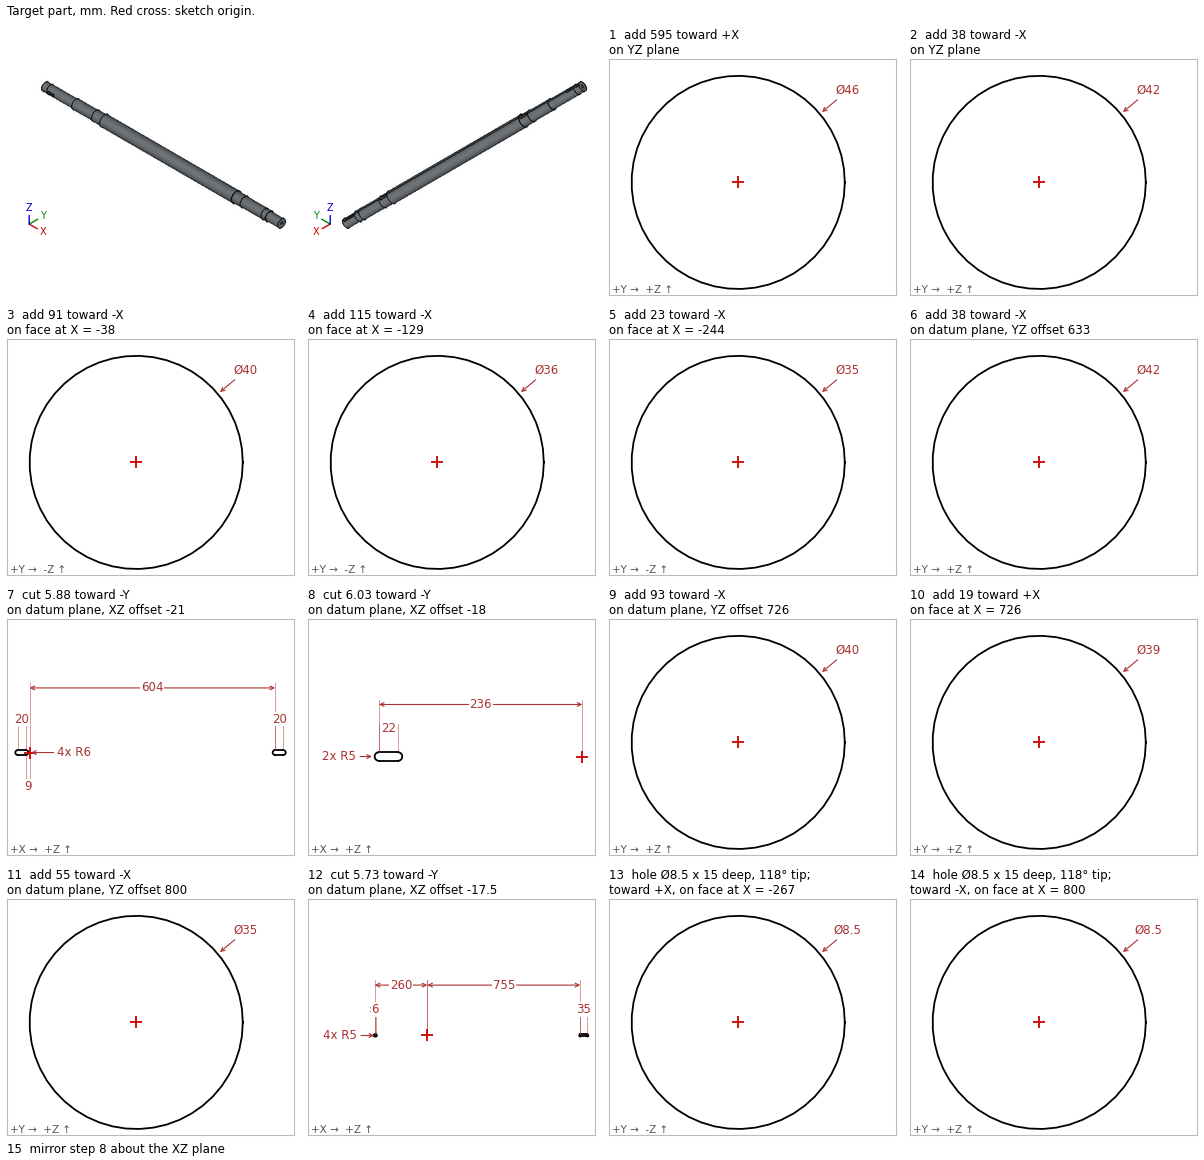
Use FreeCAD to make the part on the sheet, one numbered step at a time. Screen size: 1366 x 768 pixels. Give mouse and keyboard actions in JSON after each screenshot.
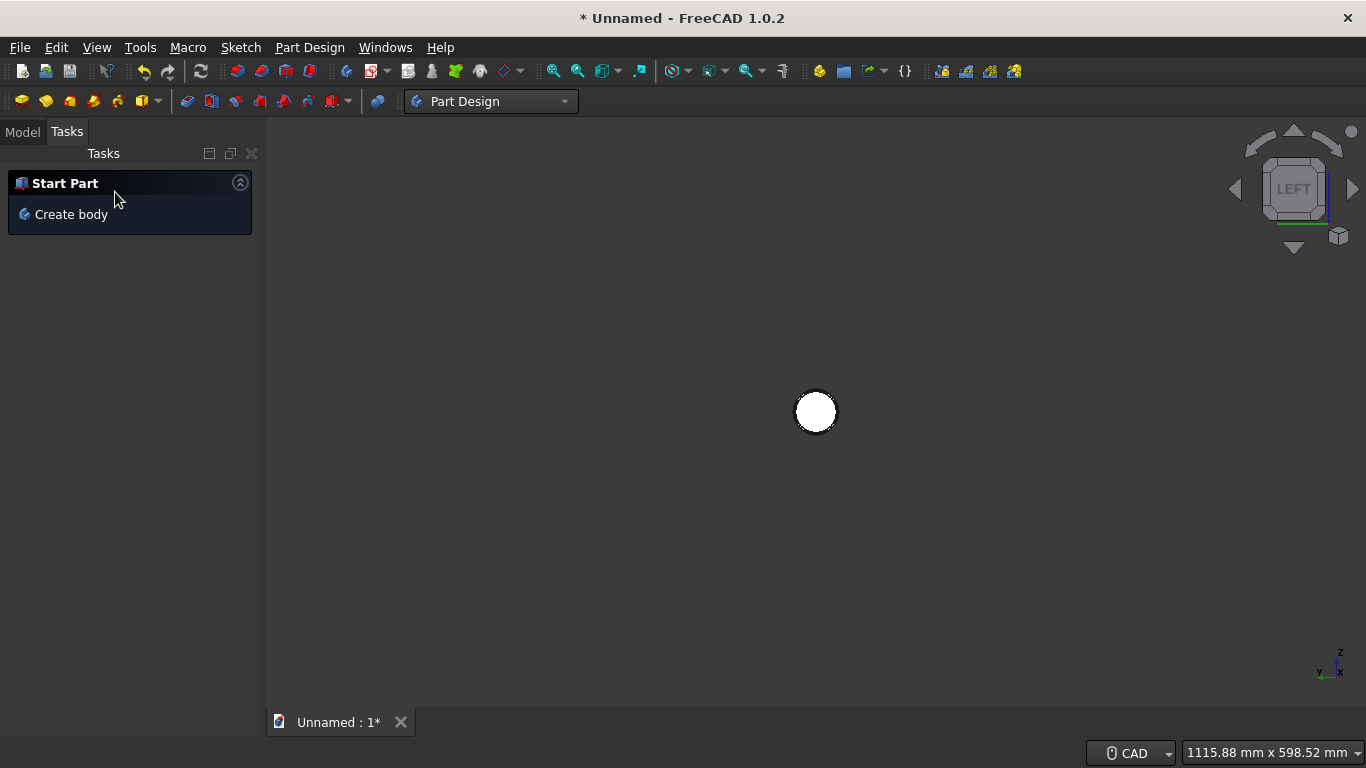
{"action": "left_click", "coordinate": [554, 72]}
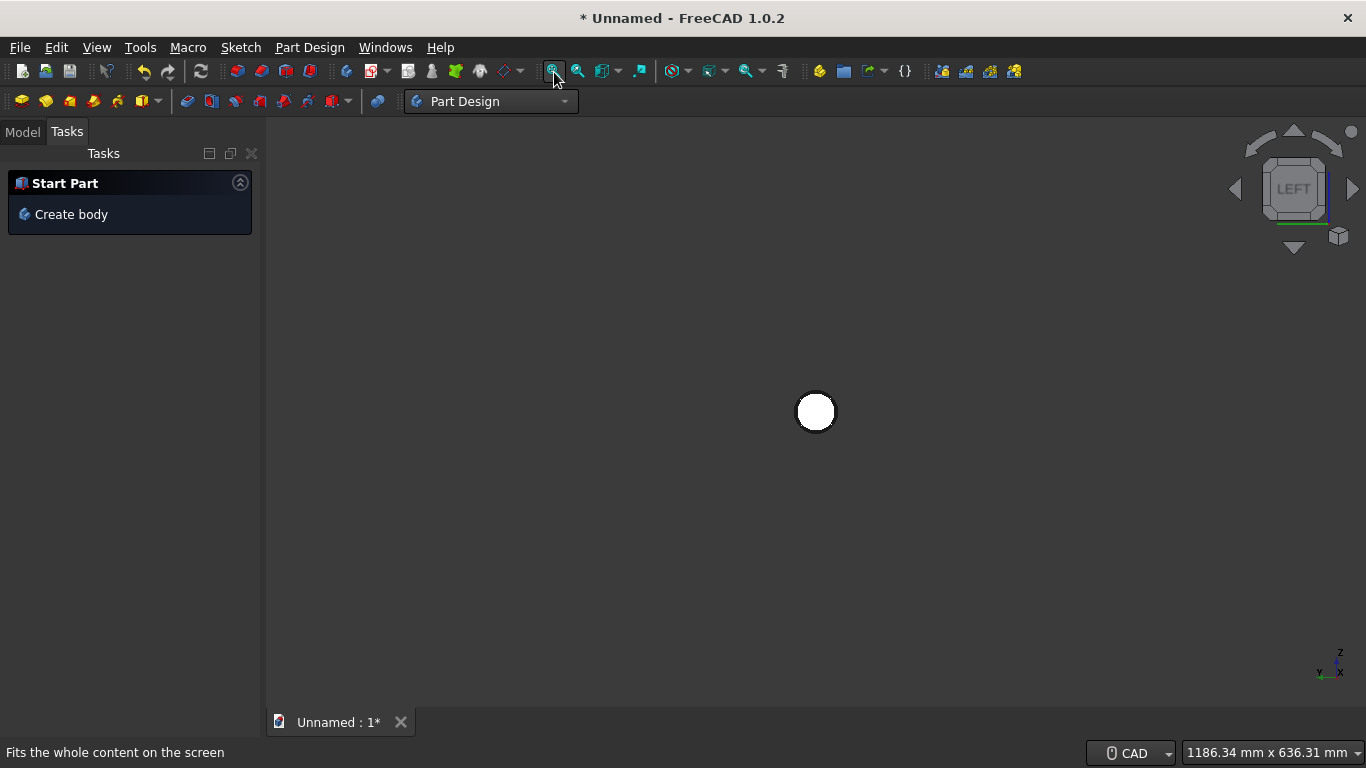
{"action": "left_click", "coordinate": [816, 411]}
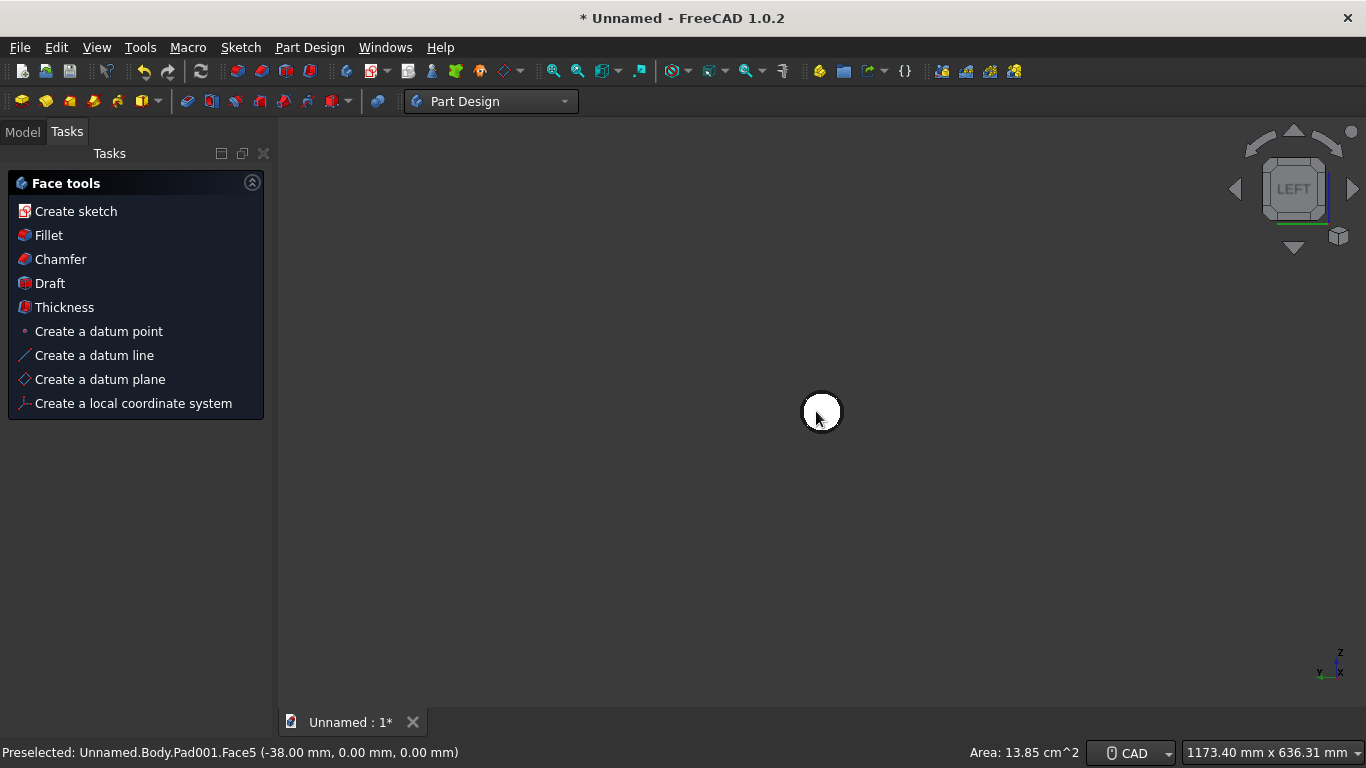
{"action": "left_click", "coordinate": [372, 72]}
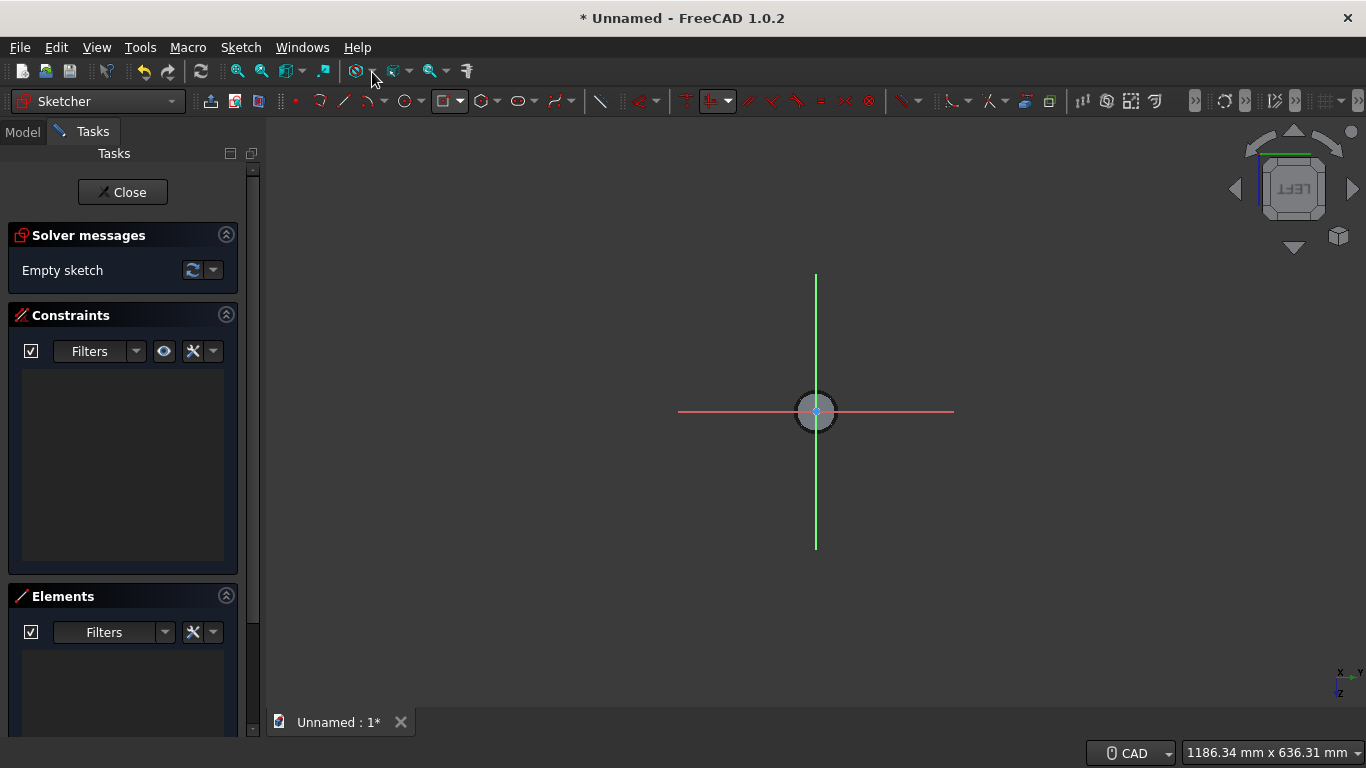
{"action": "scroll", "coordinate": [823, 412], "scroll_direction": "up", "scroll_amount": 12}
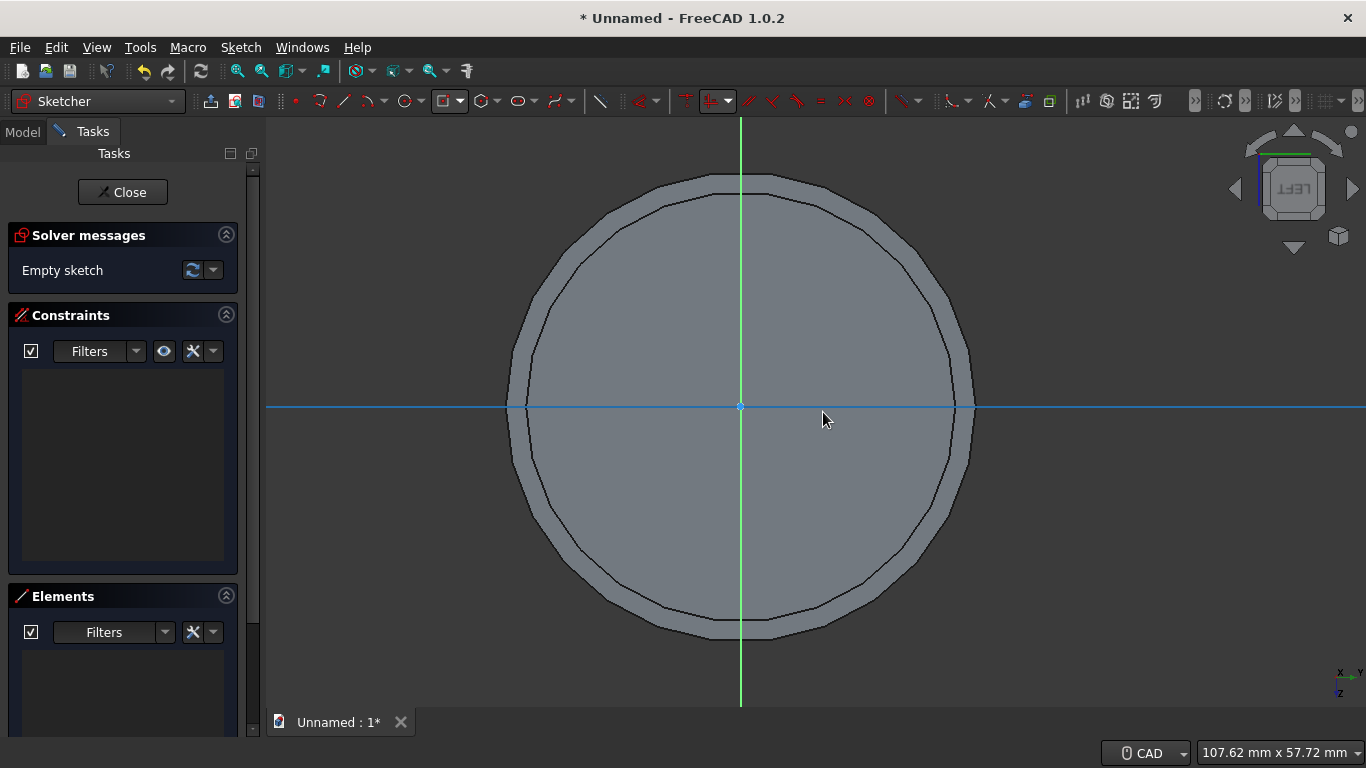
{"action": "key", "text": "g c"}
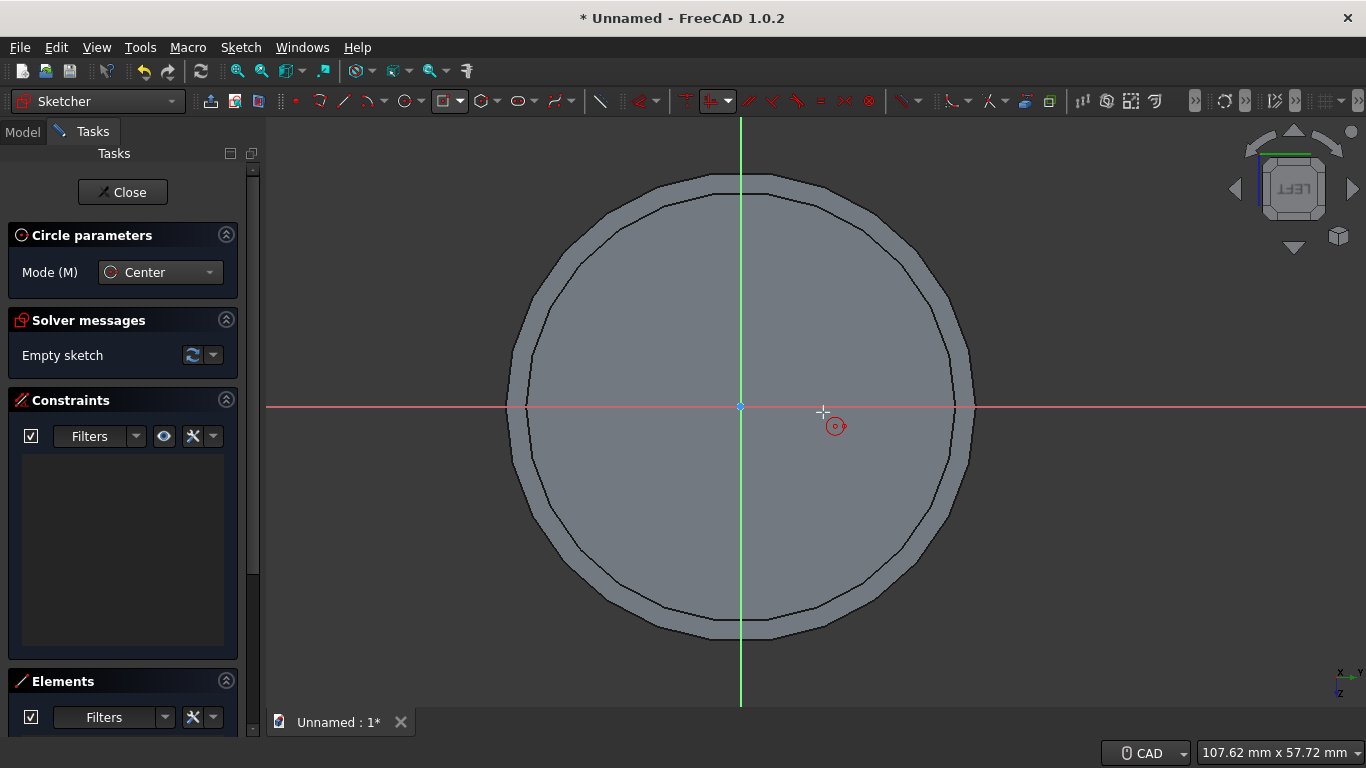
{"action": "left_click", "coordinate": [741, 407]}
{"action": "mouse_move", "coordinate": [885, 262]}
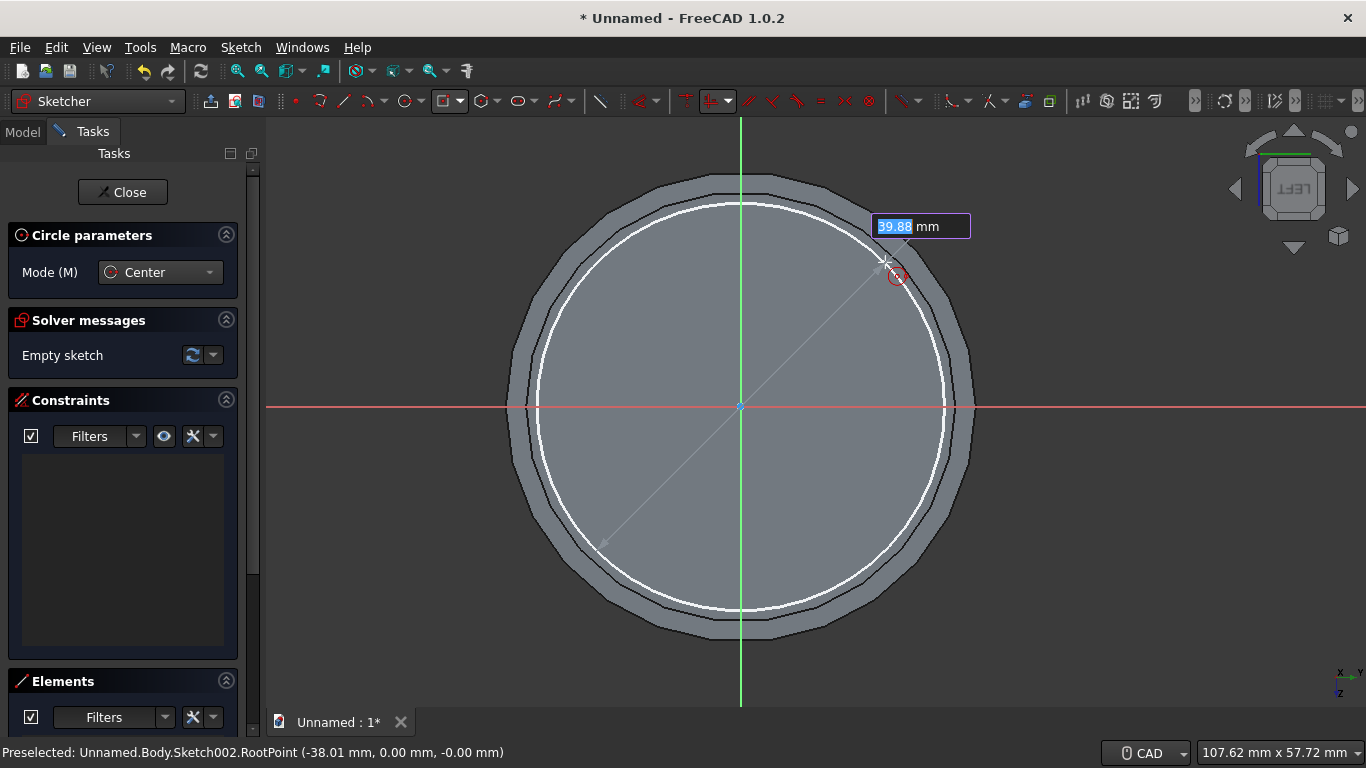
{"action": "type", "text": "40"}
{"action": "key", "text": "Return"}
{"action": "key", "text": "Escape"}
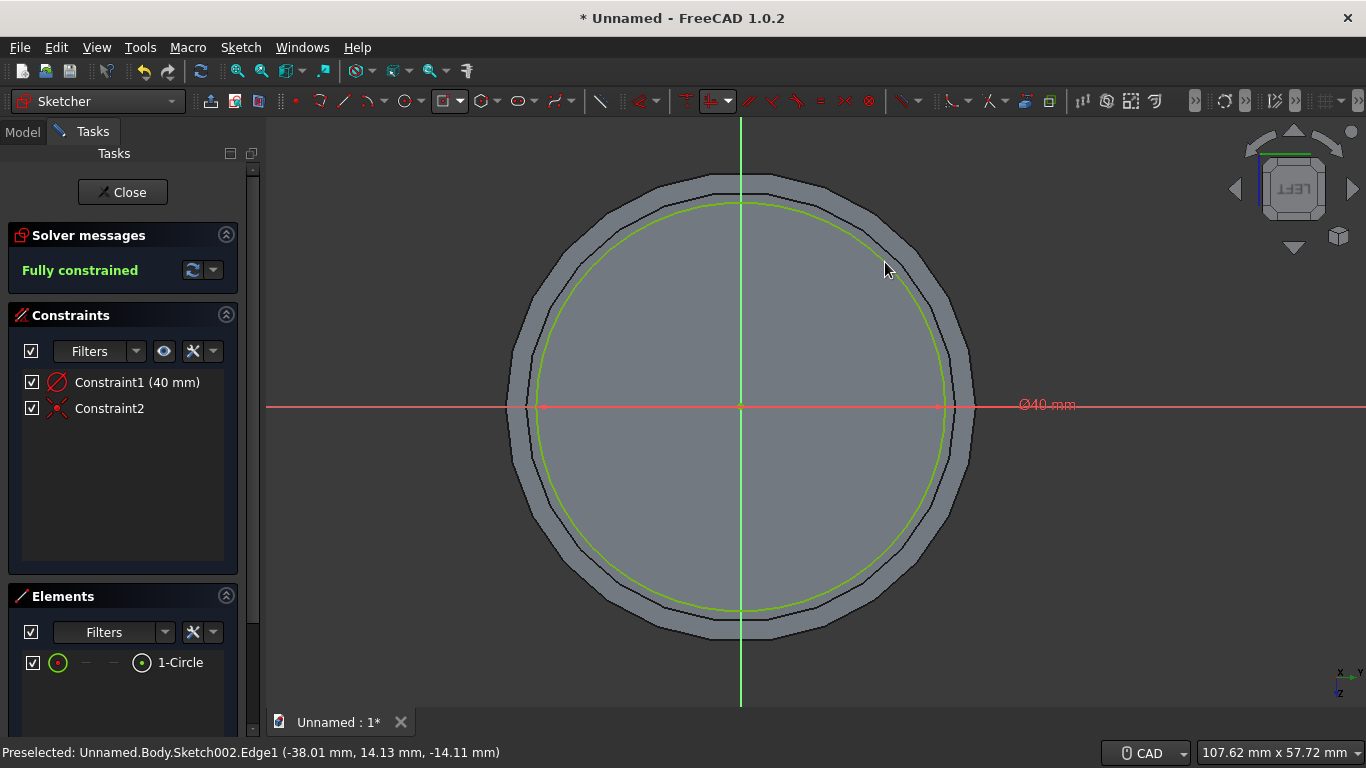
{"action": "left_click", "coordinate": [123, 192]}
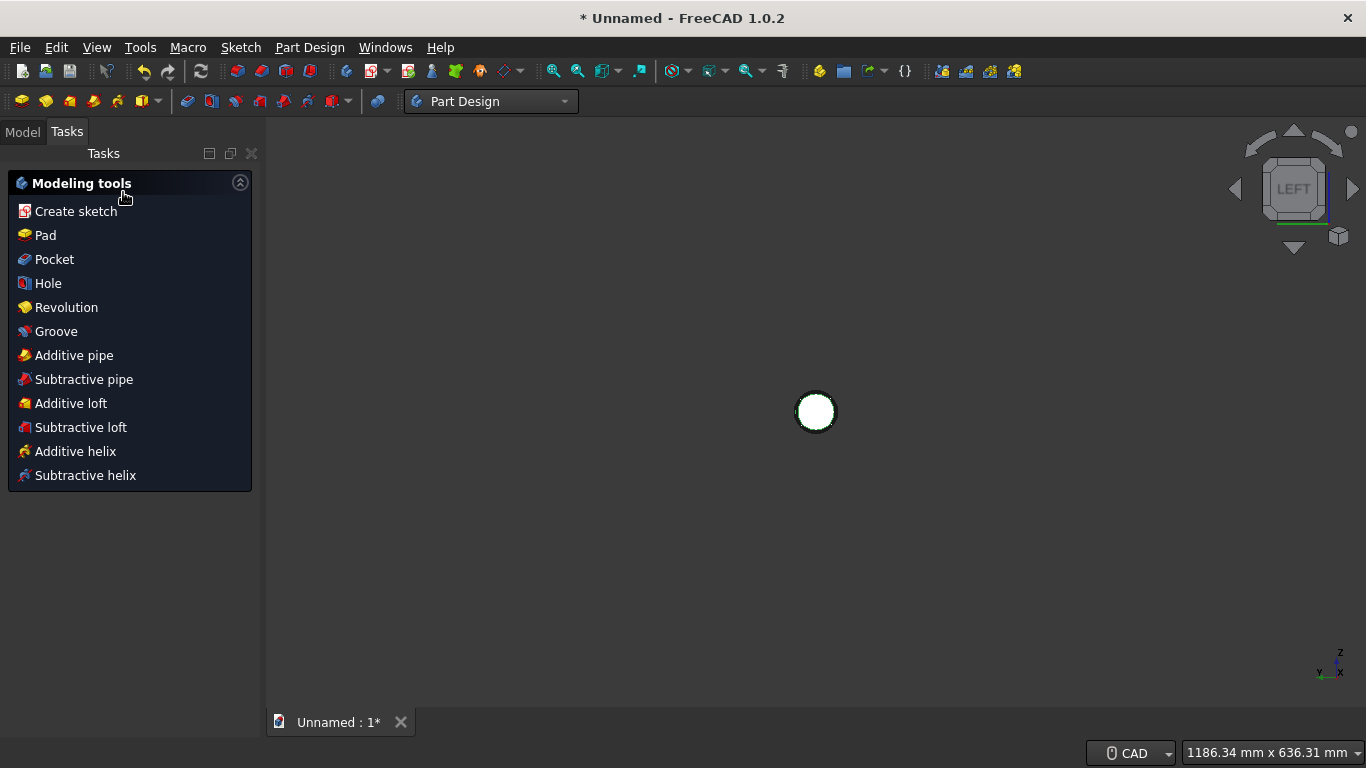
{"action": "left_click", "coordinate": [22, 102]}